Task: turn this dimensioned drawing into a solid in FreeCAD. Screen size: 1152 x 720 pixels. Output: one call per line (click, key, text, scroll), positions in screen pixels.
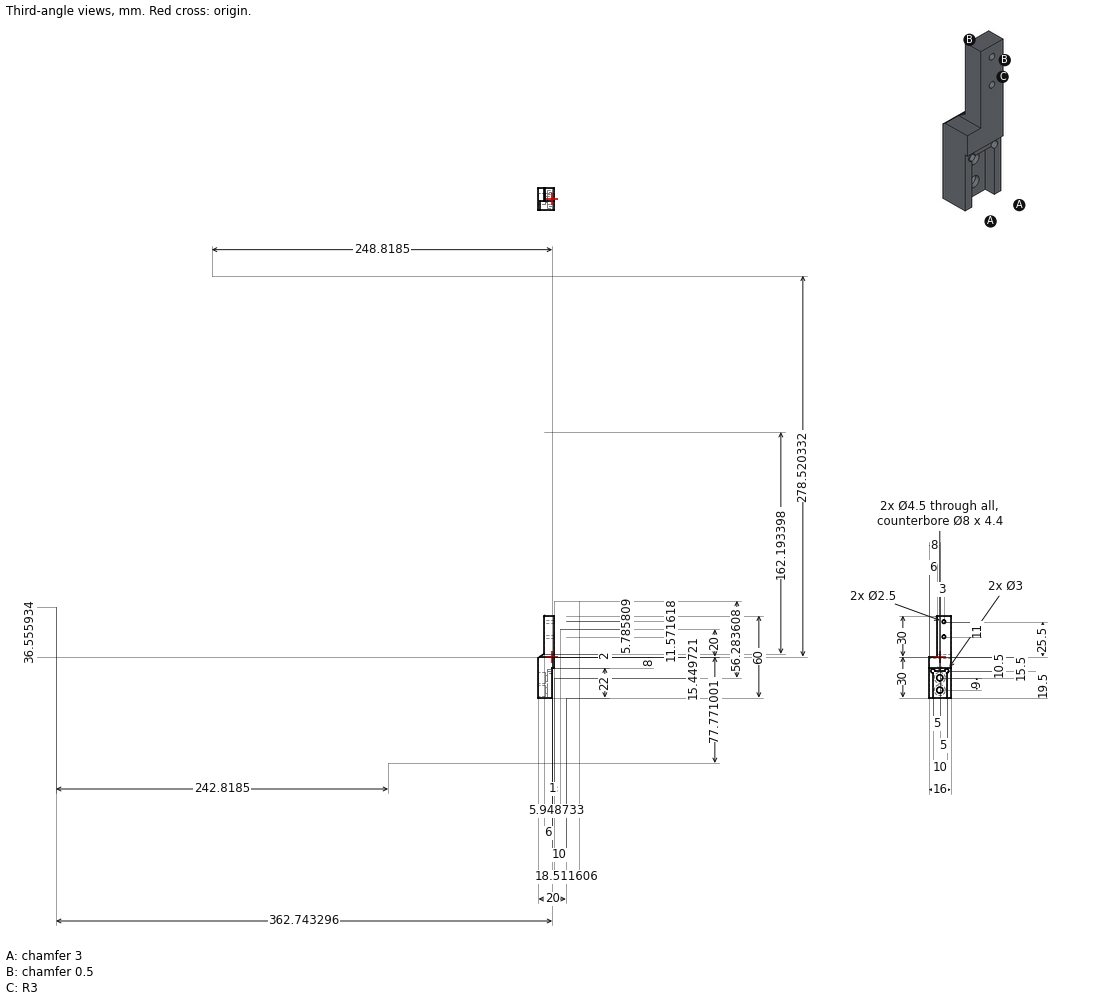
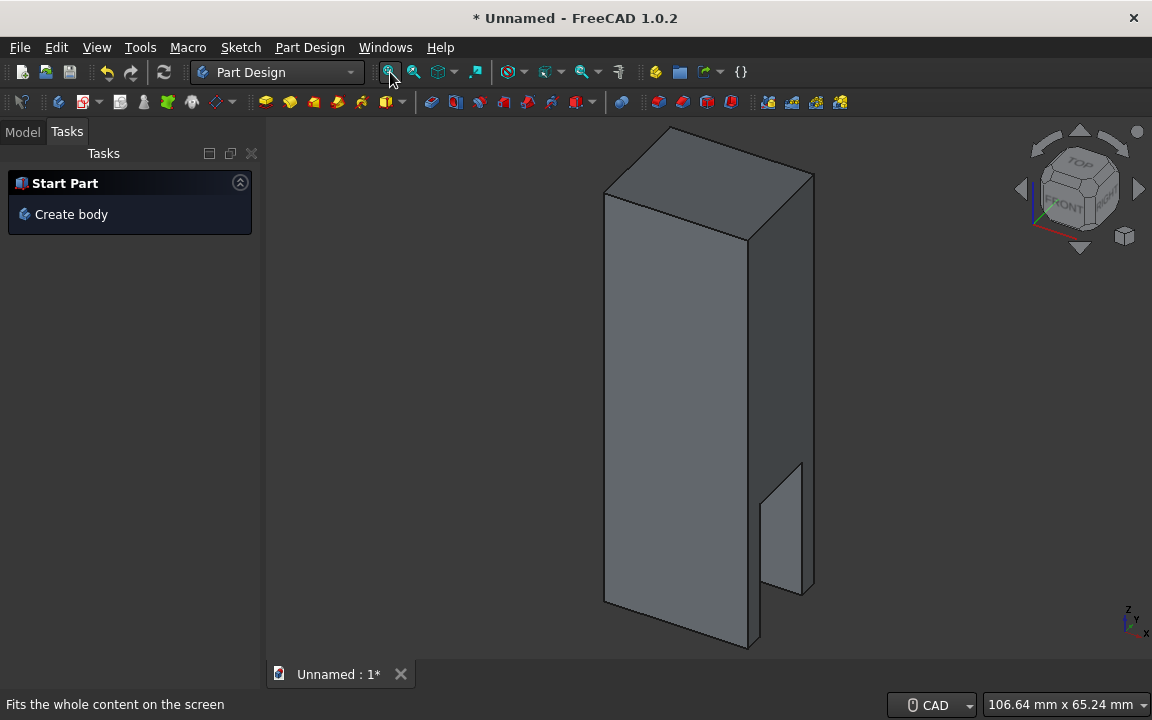
key(0)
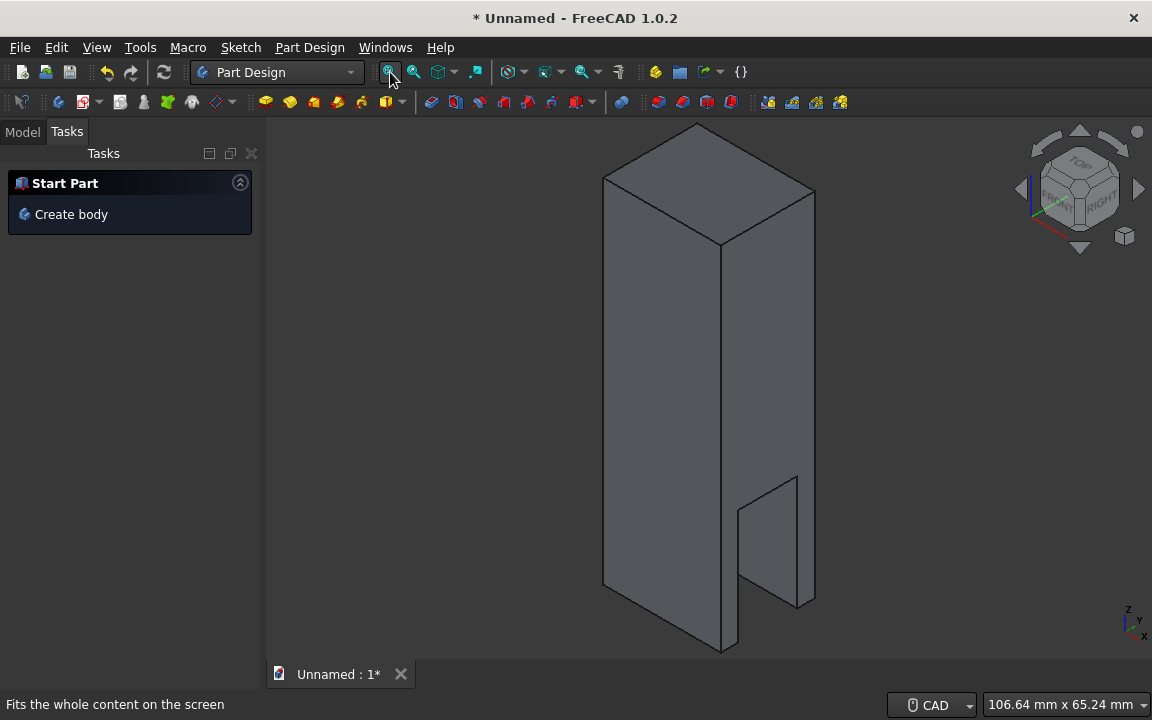
key(2)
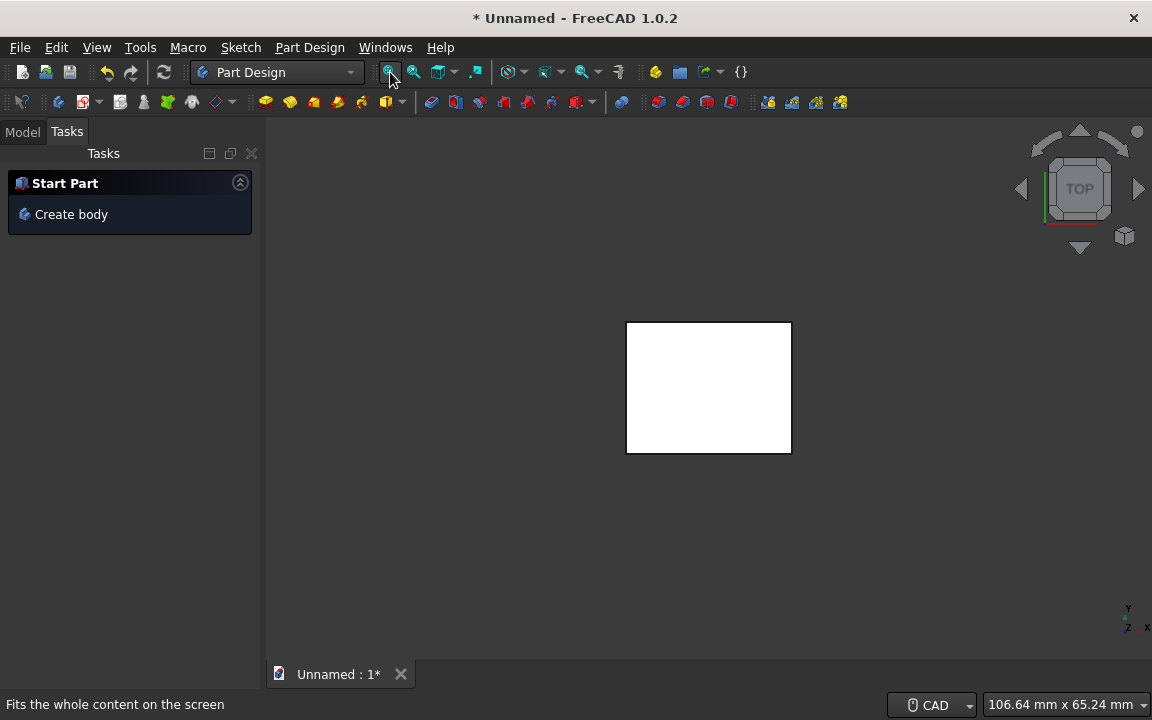
key(v)
key(f)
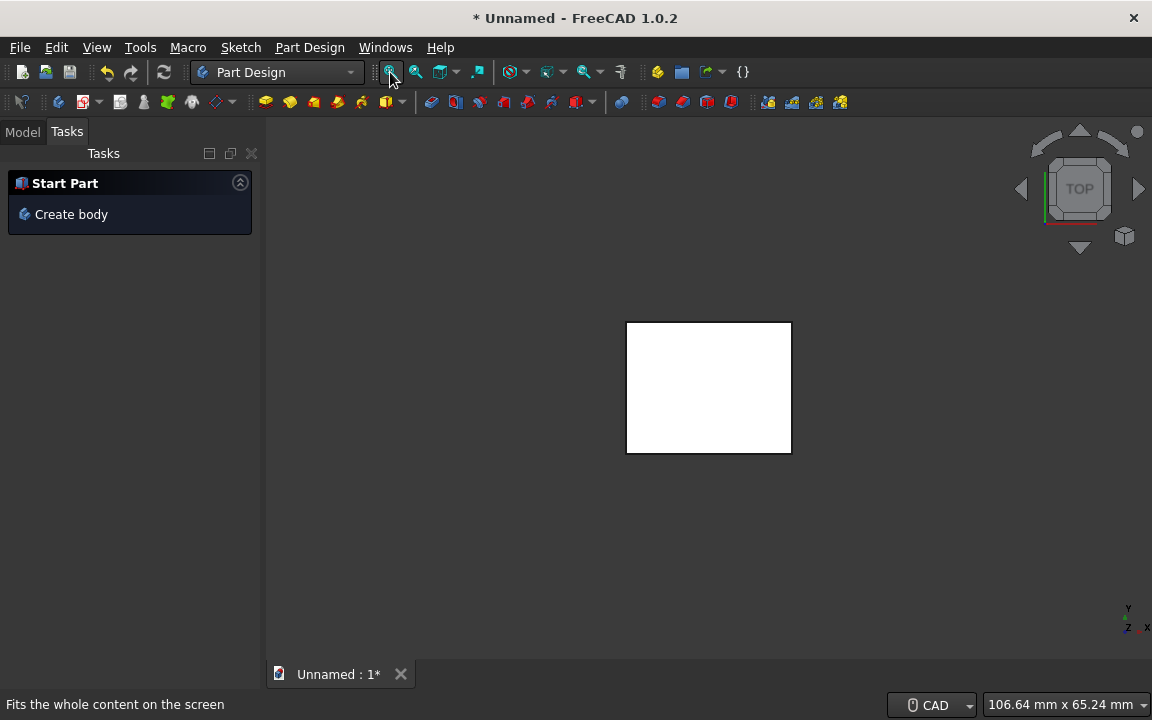
key(1)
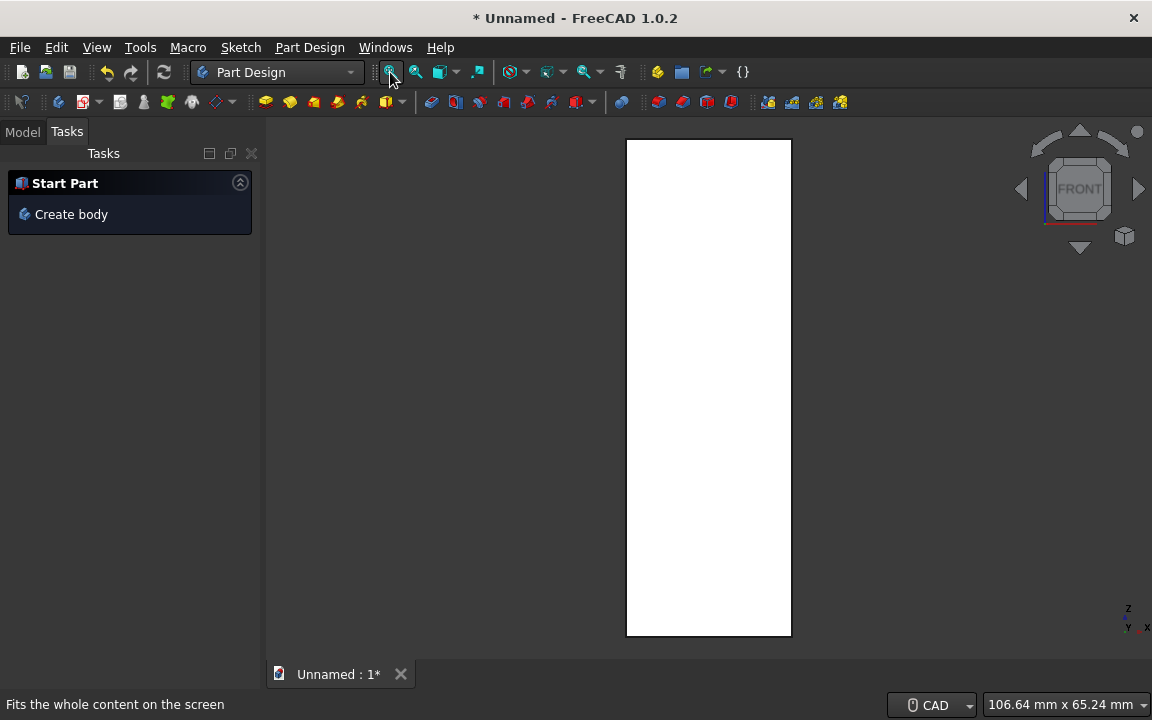
key(3)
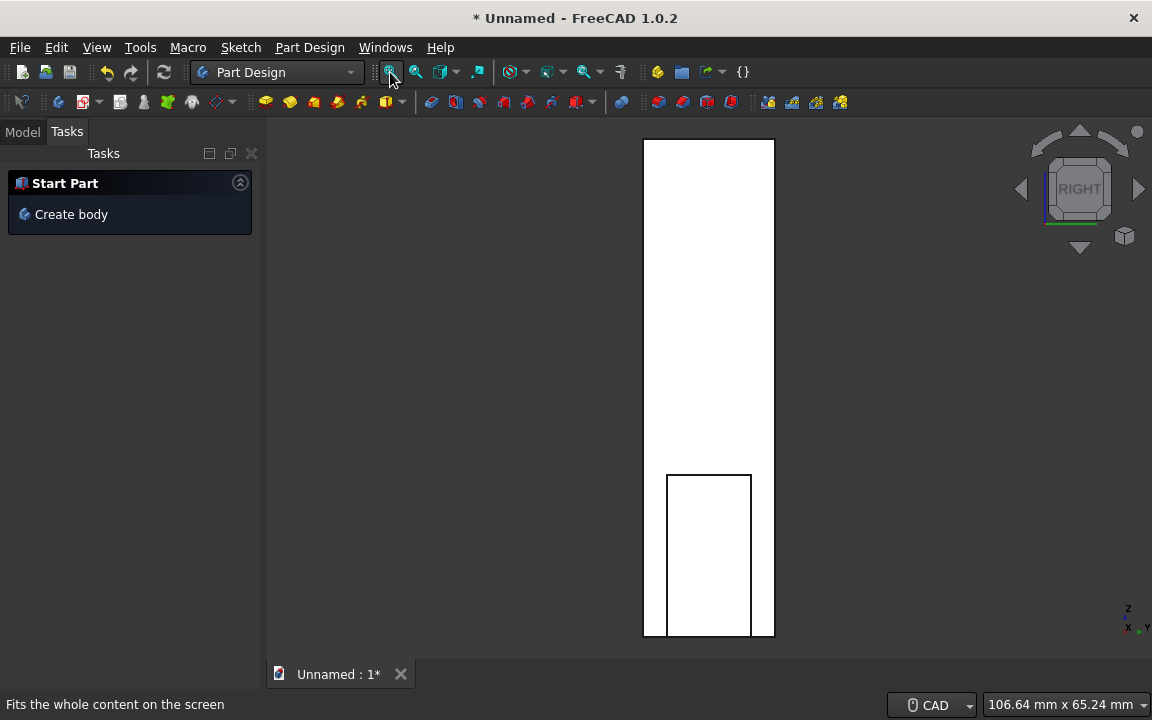
key(5)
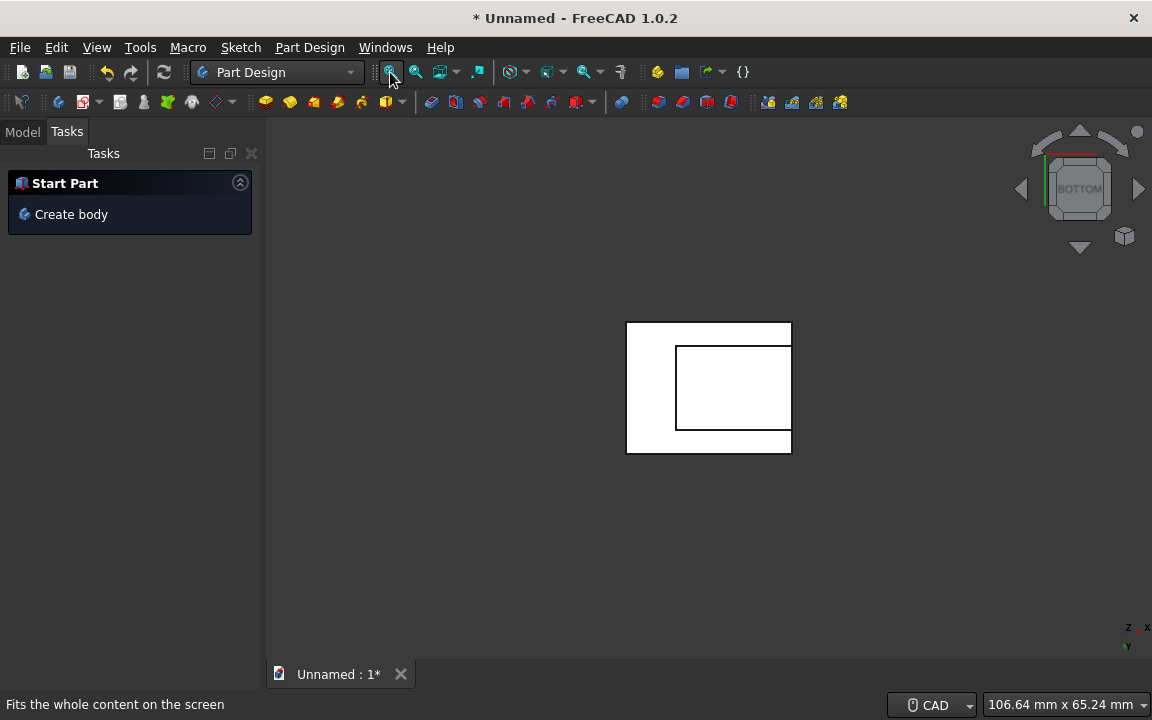
click(392, 72)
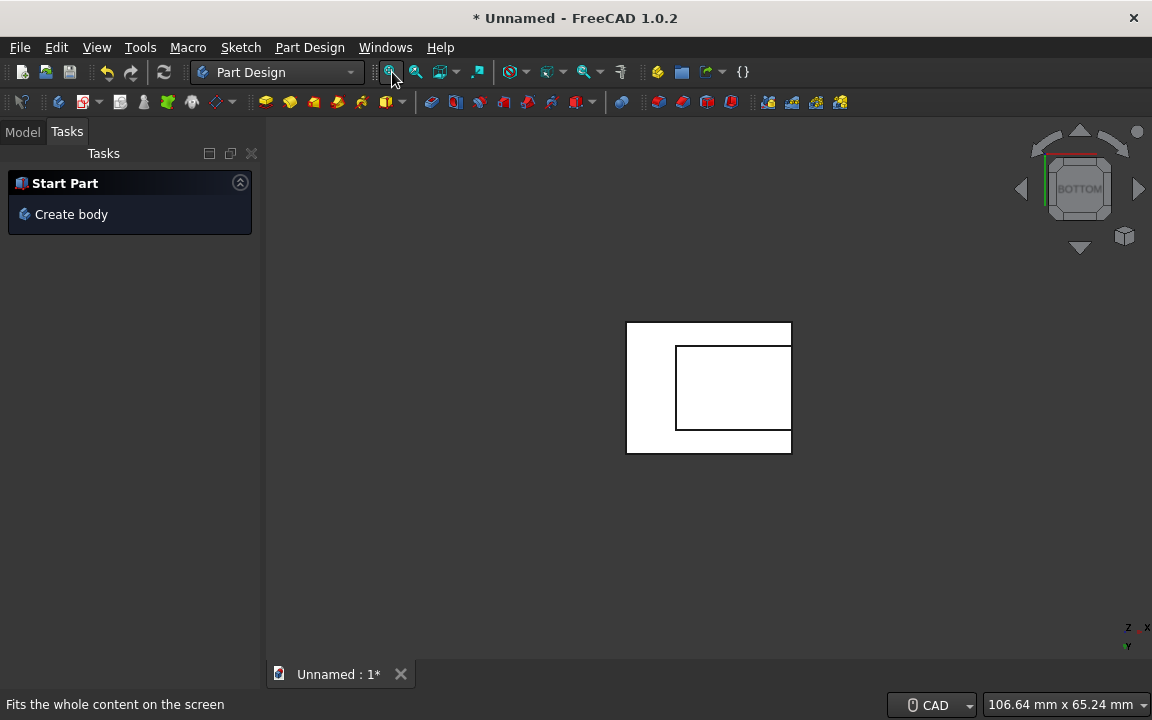
click(792, 333)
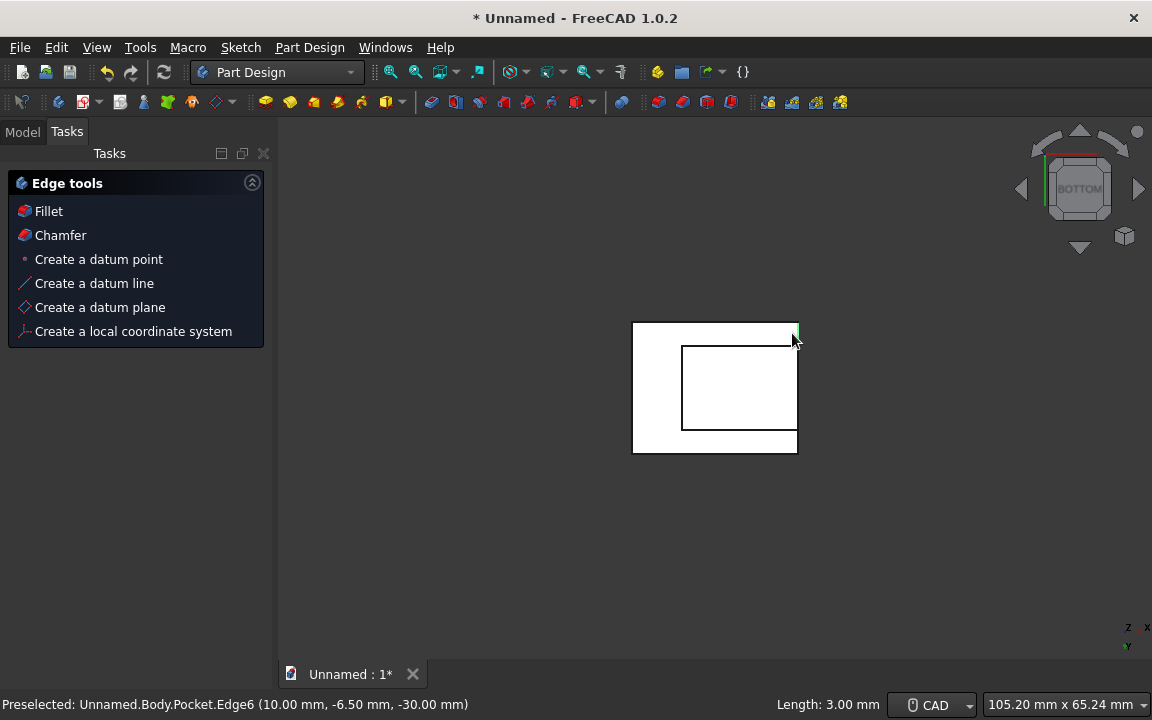
click(798, 441, ctrl)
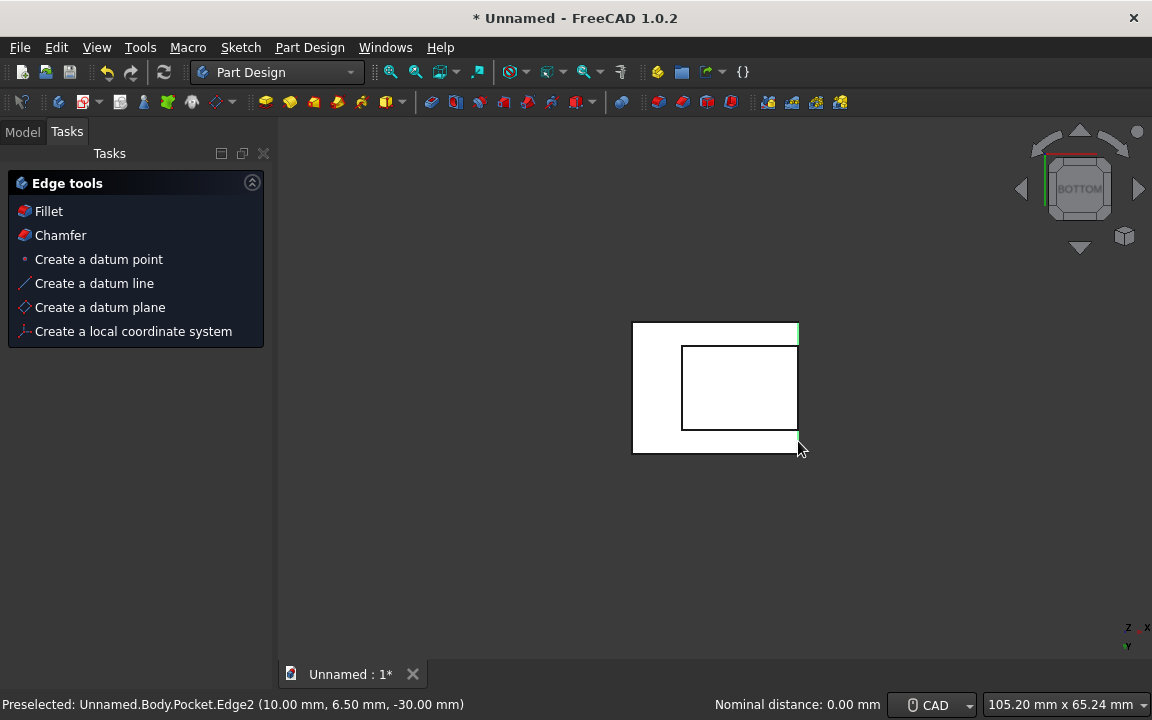
click(684, 102)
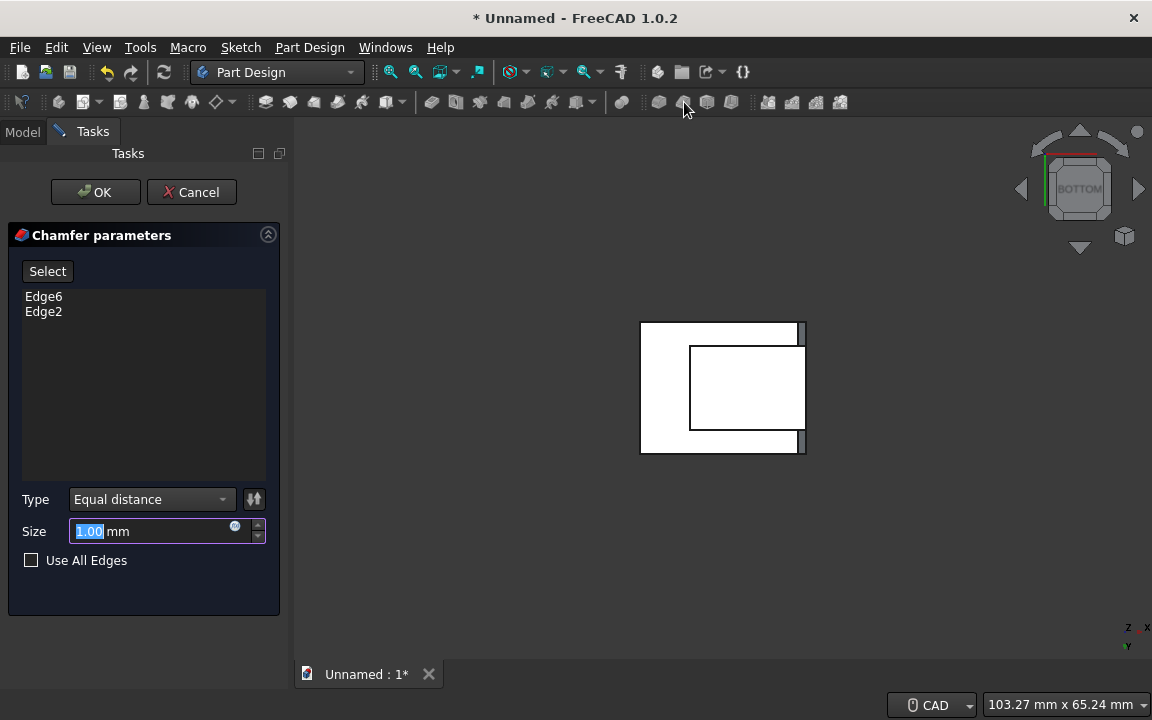
text(3)
key(Tab)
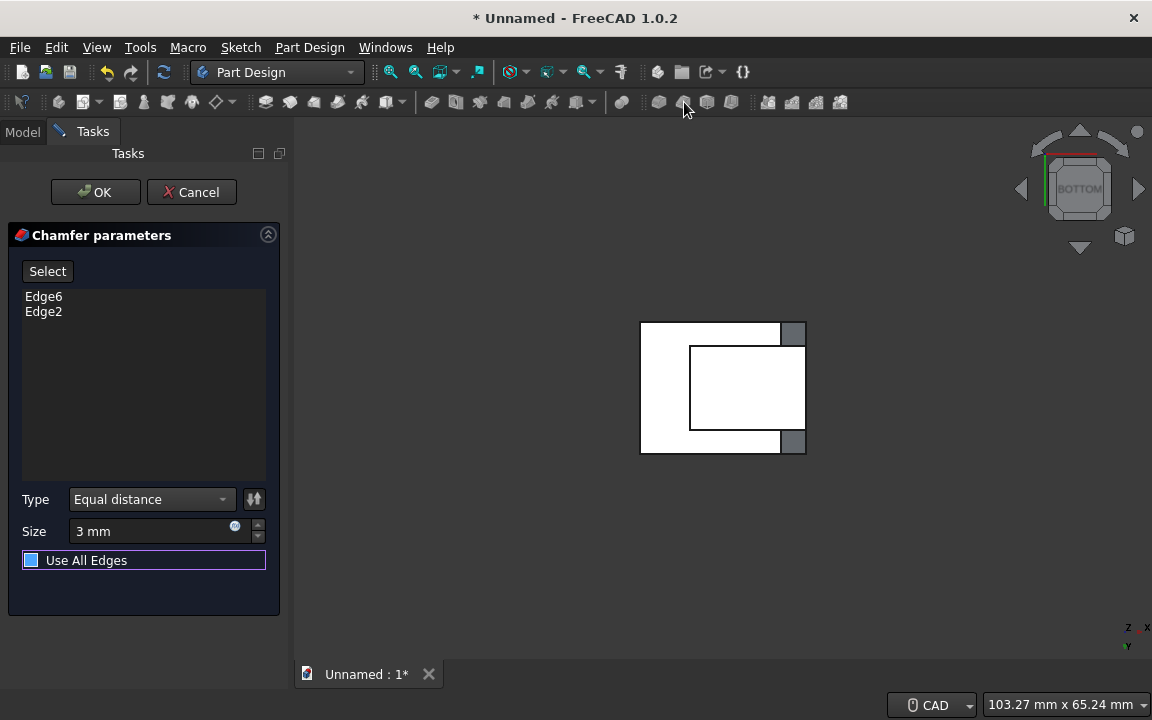
click(96, 192)